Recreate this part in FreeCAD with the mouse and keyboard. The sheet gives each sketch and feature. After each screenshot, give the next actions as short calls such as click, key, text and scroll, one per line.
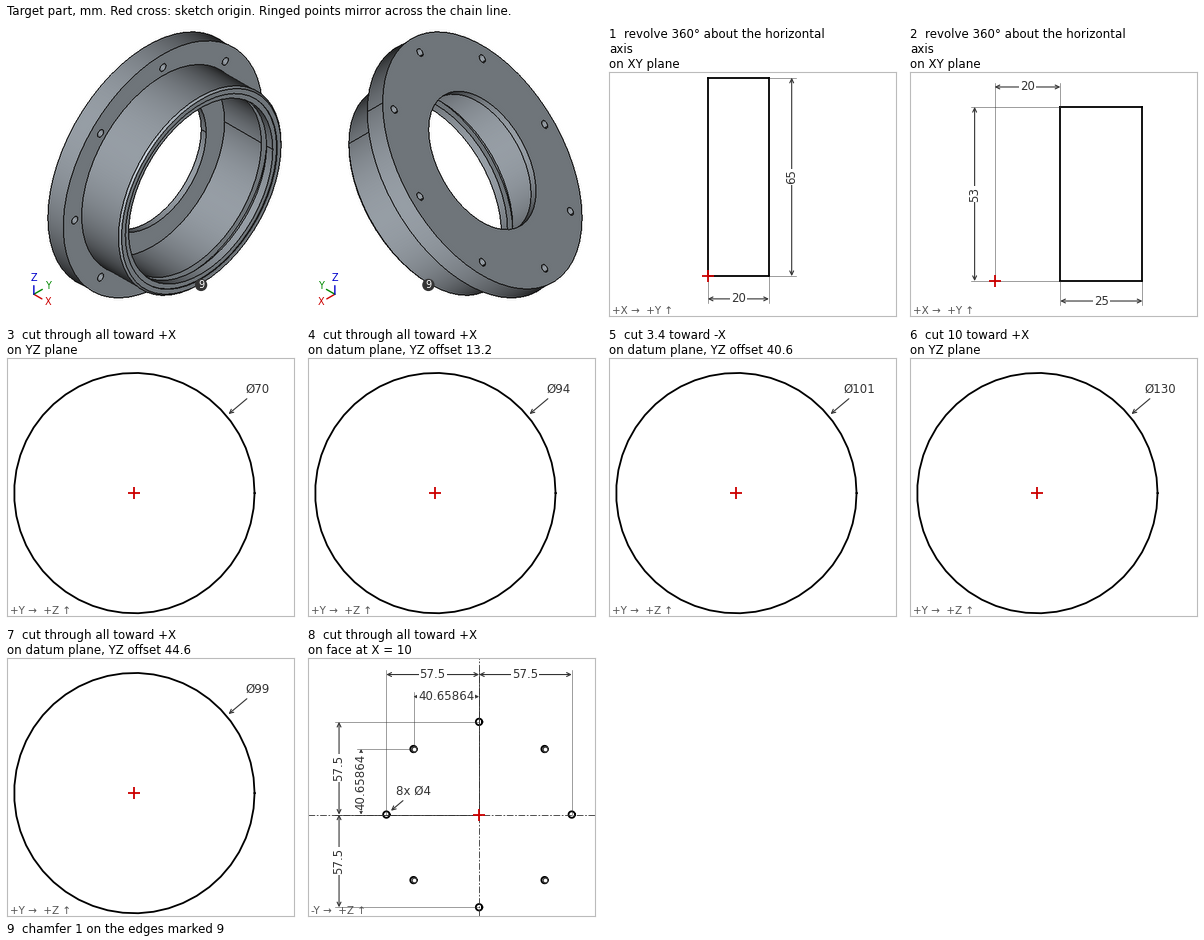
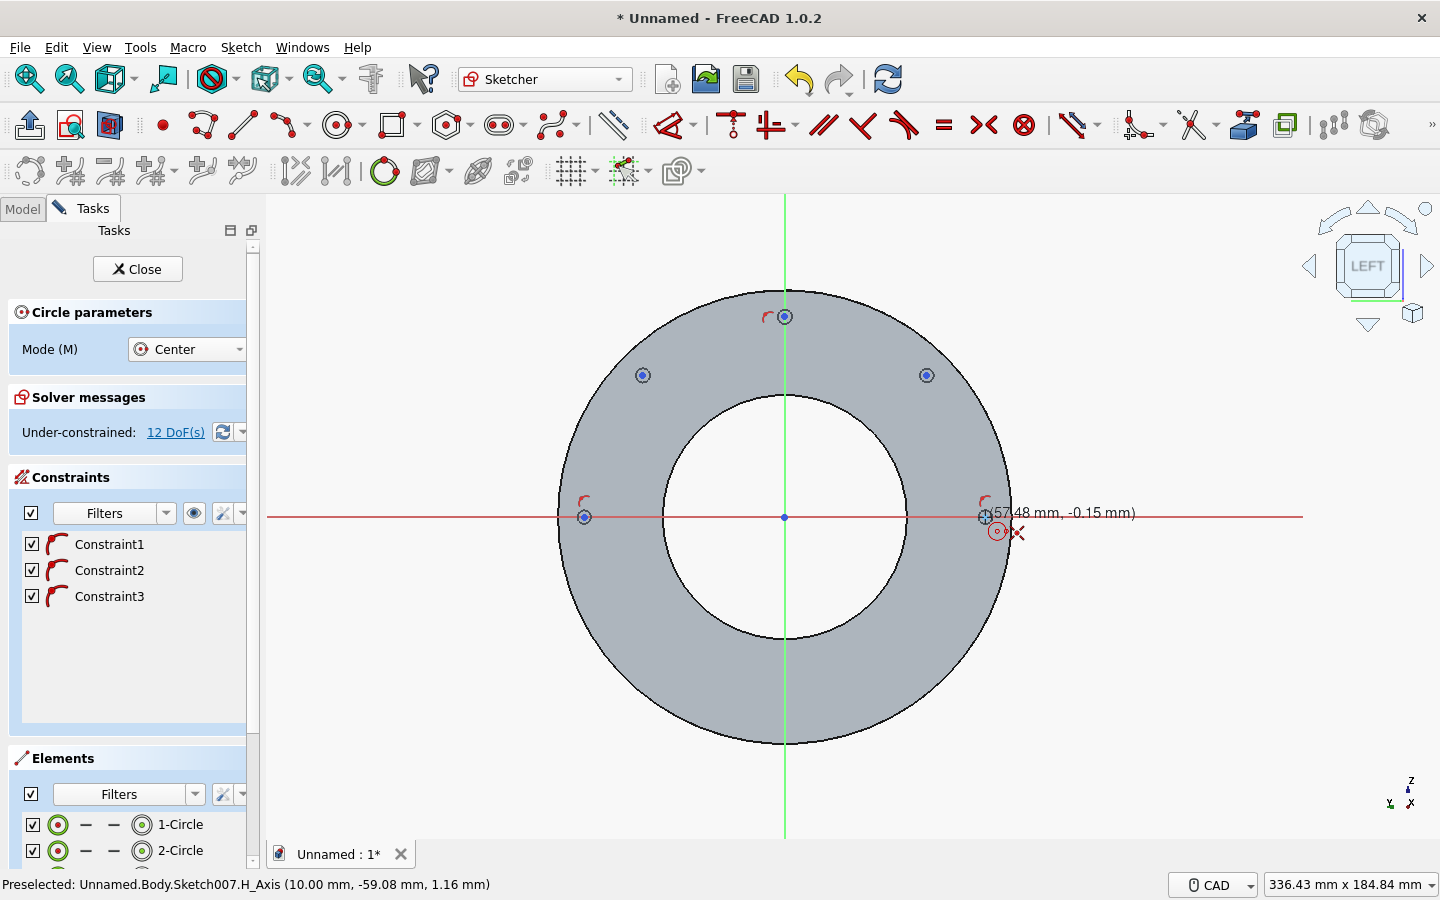
scroll(927, 659, up, 6)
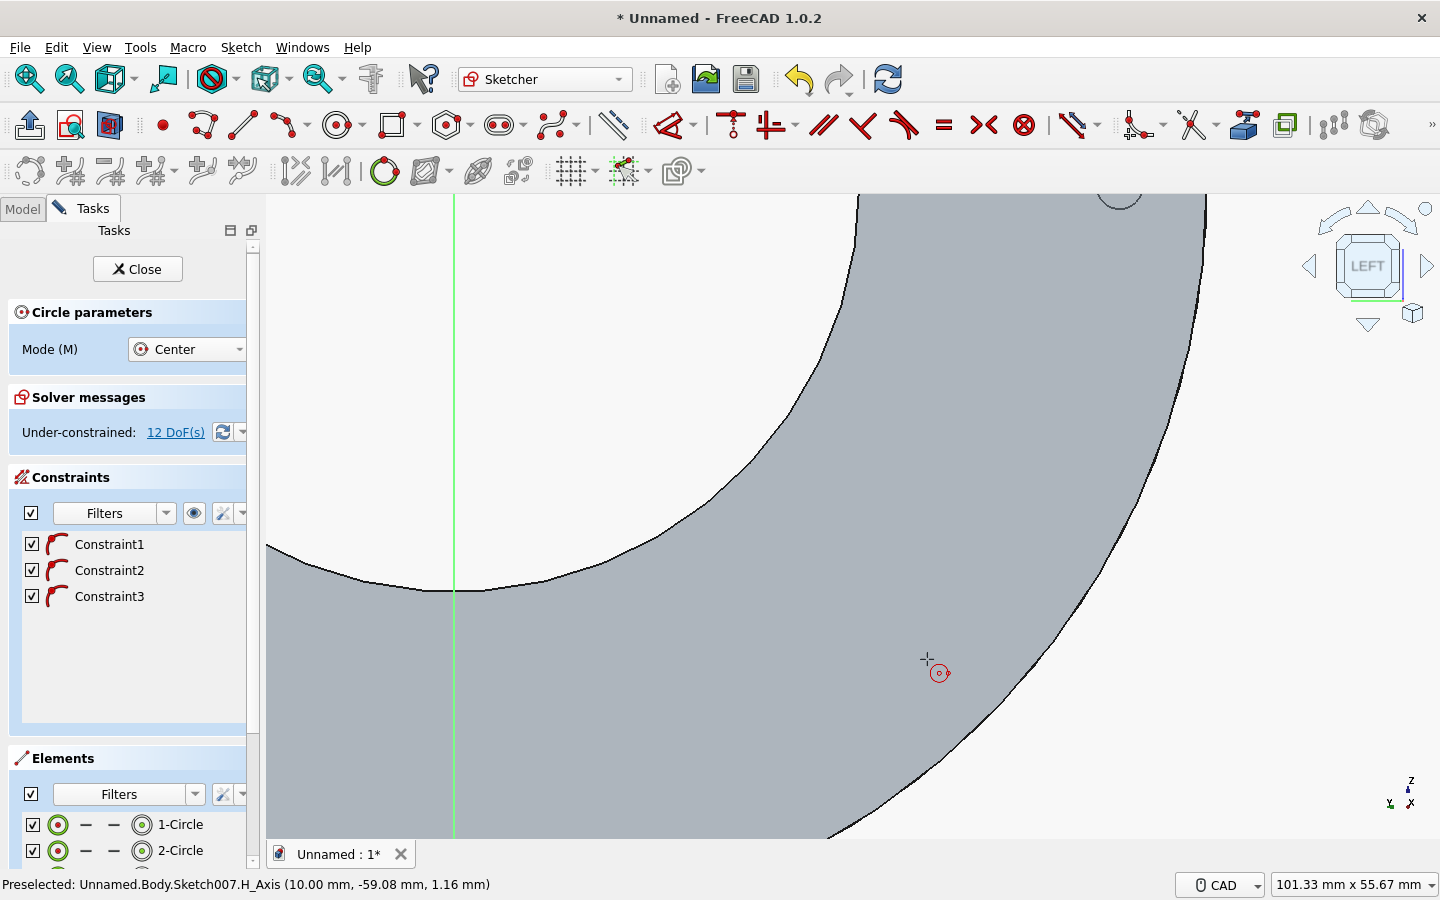
click(925, 657)
click(941, 641)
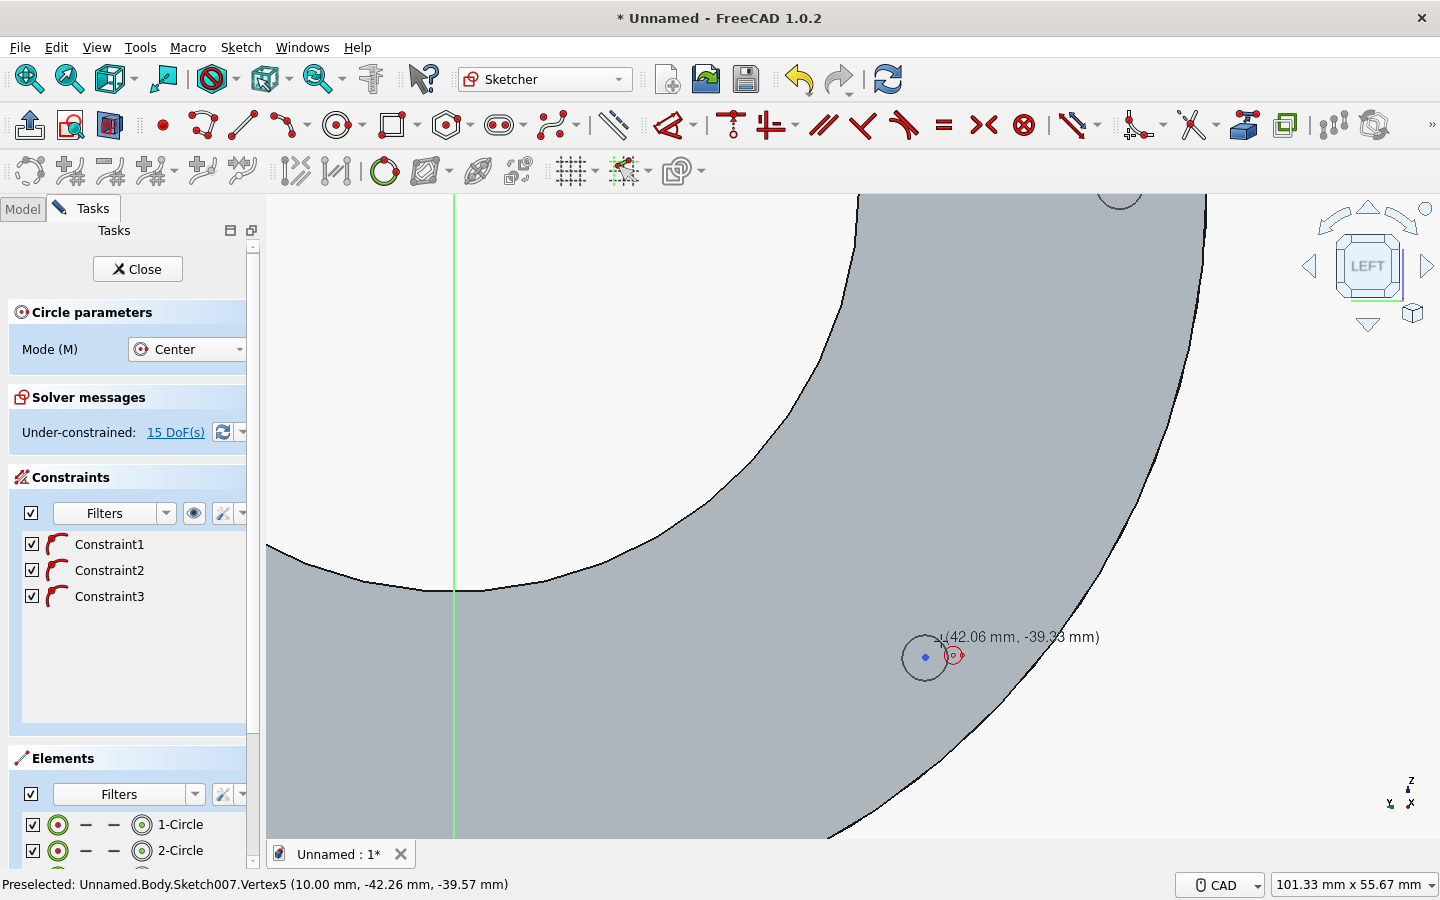
scroll(927, 659, down, 6)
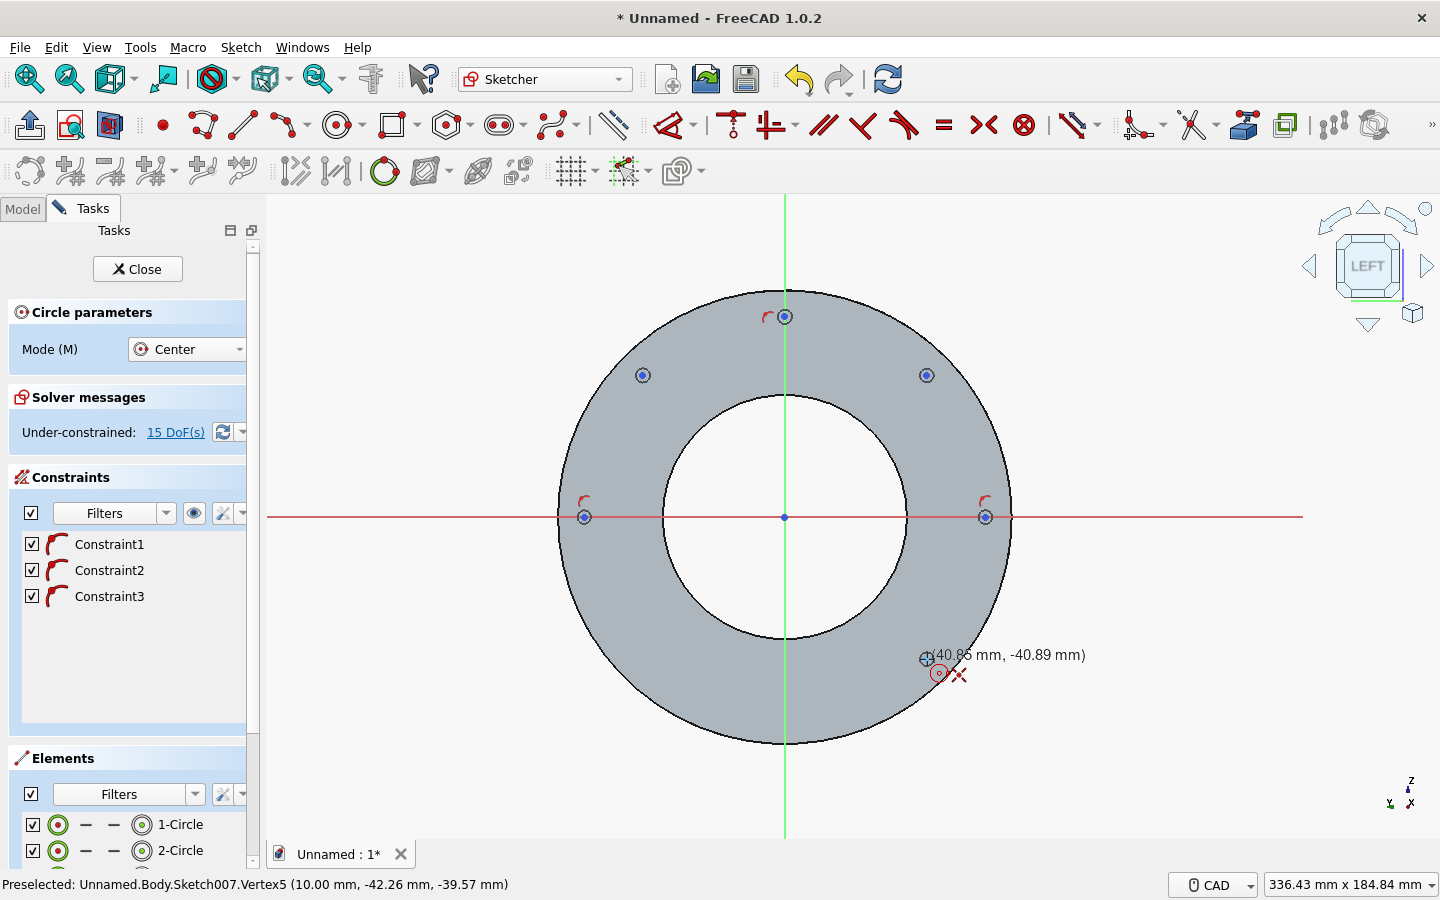
scroll(785, 718, up, 6)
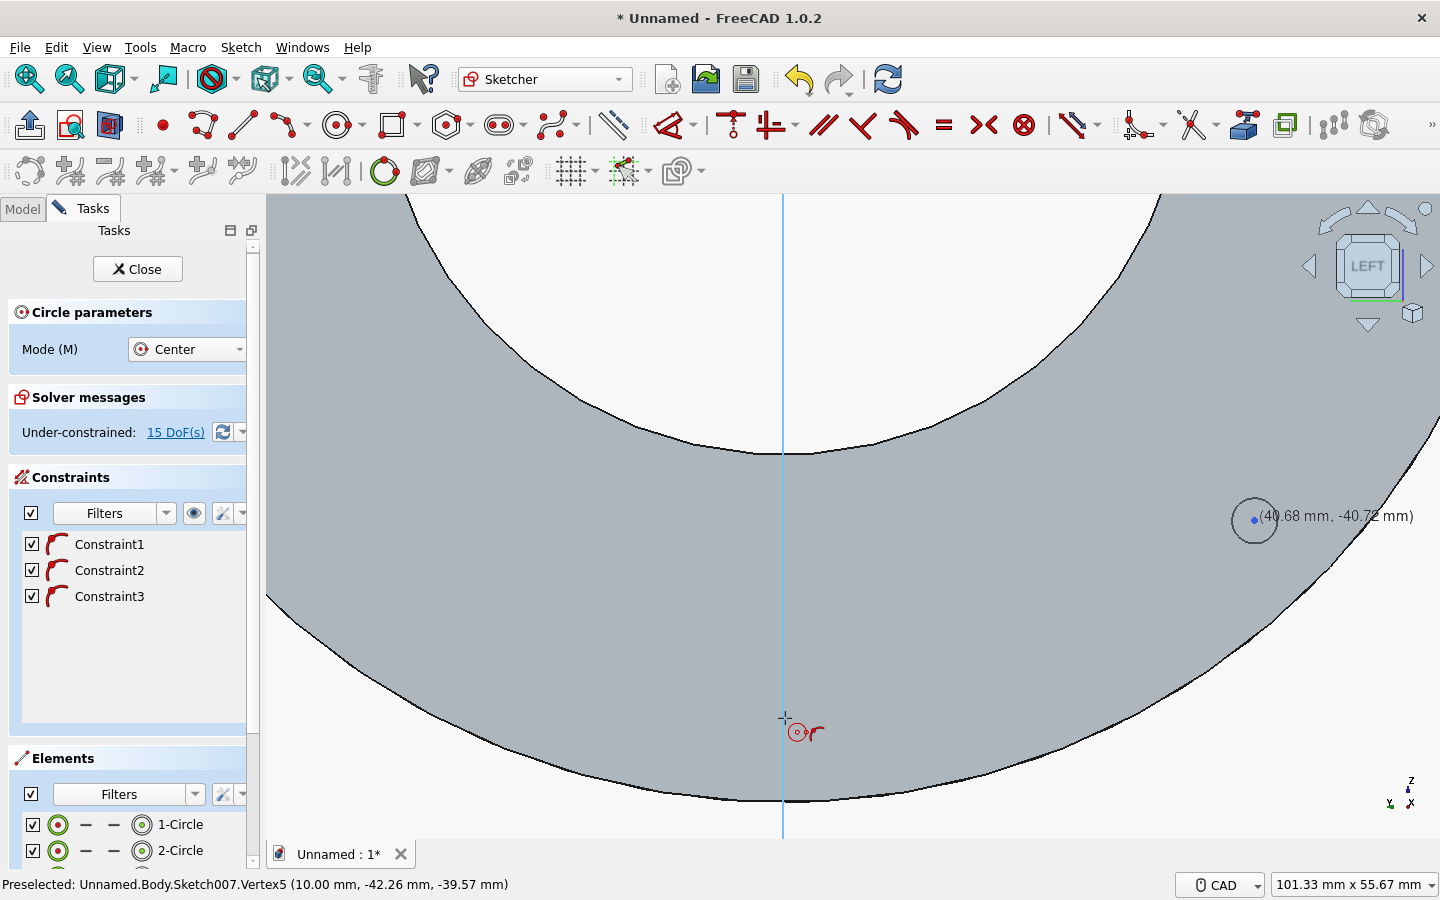
click(783, 715)
click(800, 699)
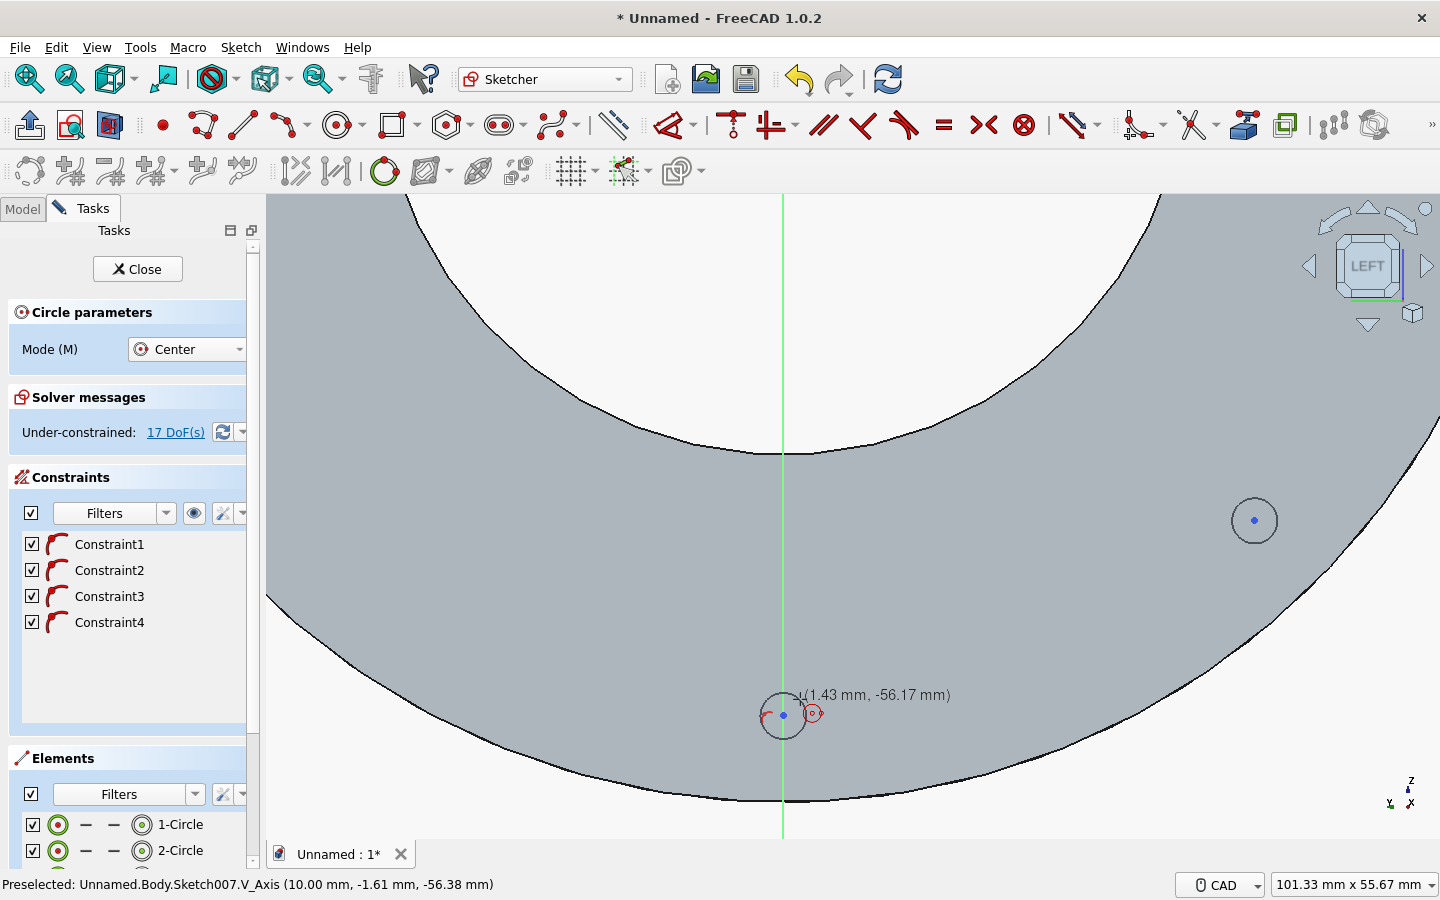
click(312, 520)
click(329, 504)
key(Escape)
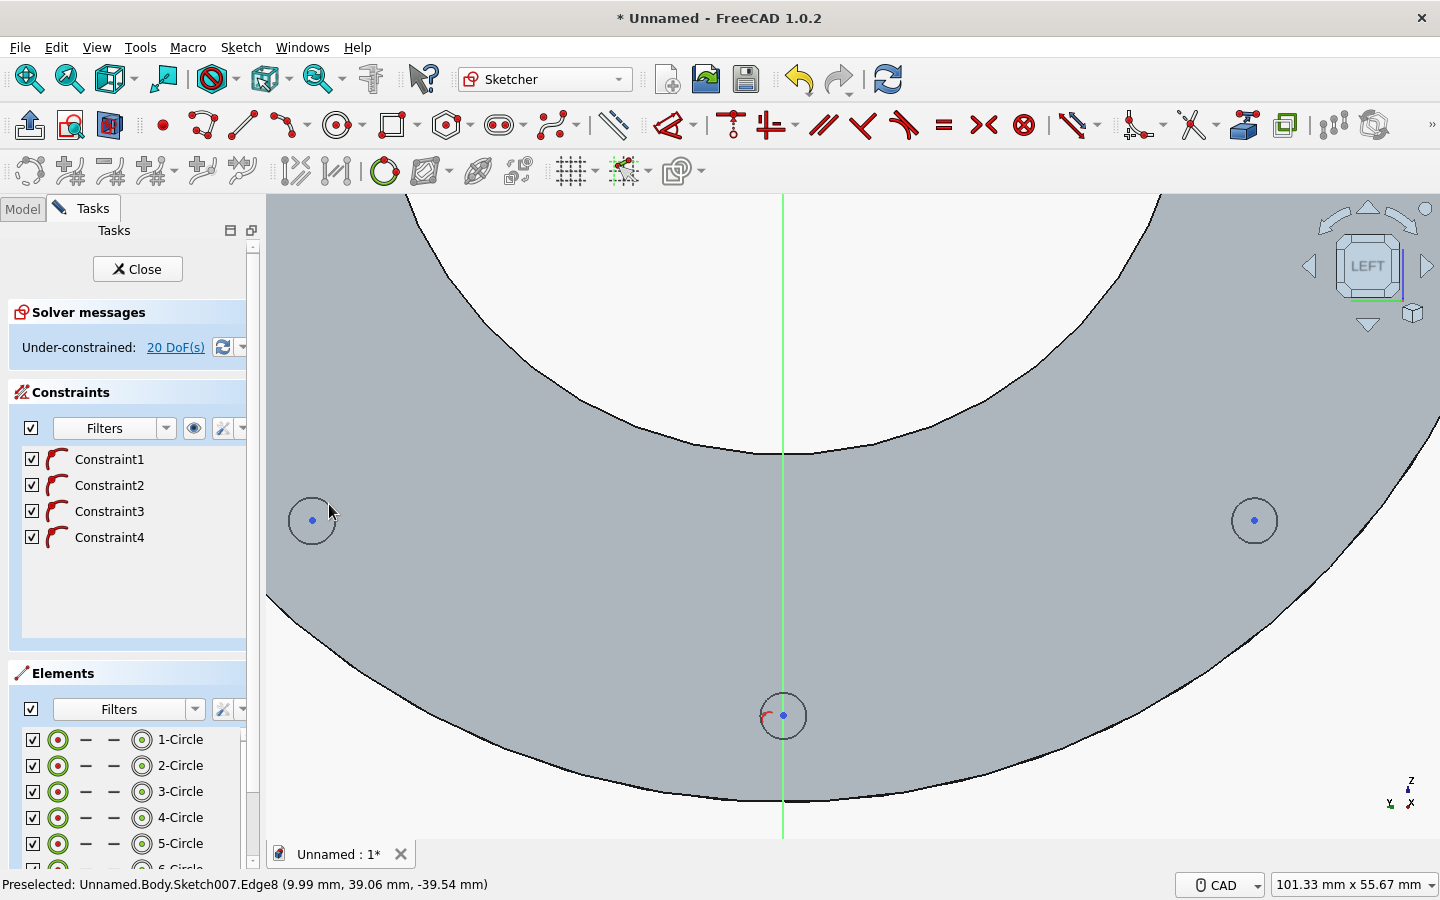
scroll(785, 718, down, 6)